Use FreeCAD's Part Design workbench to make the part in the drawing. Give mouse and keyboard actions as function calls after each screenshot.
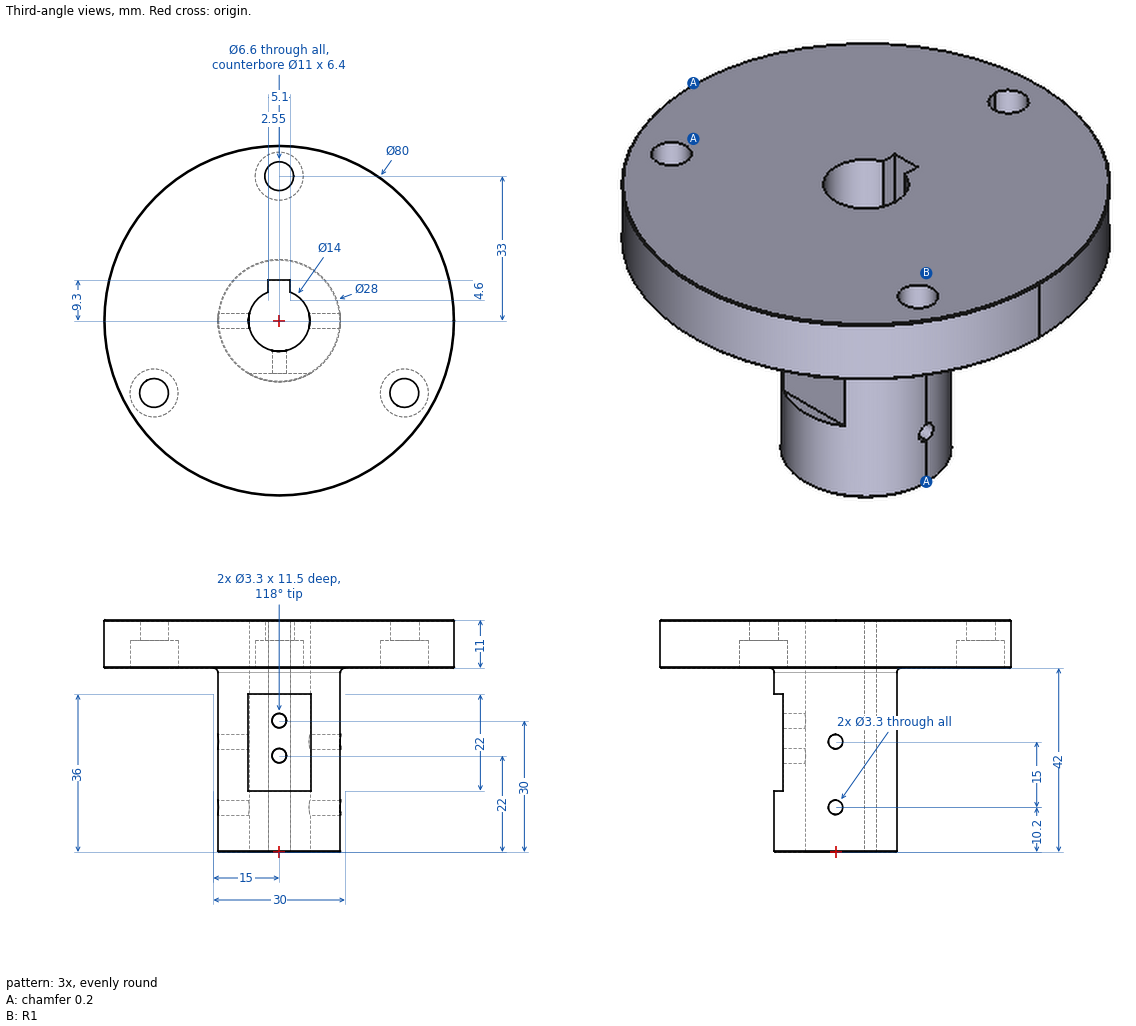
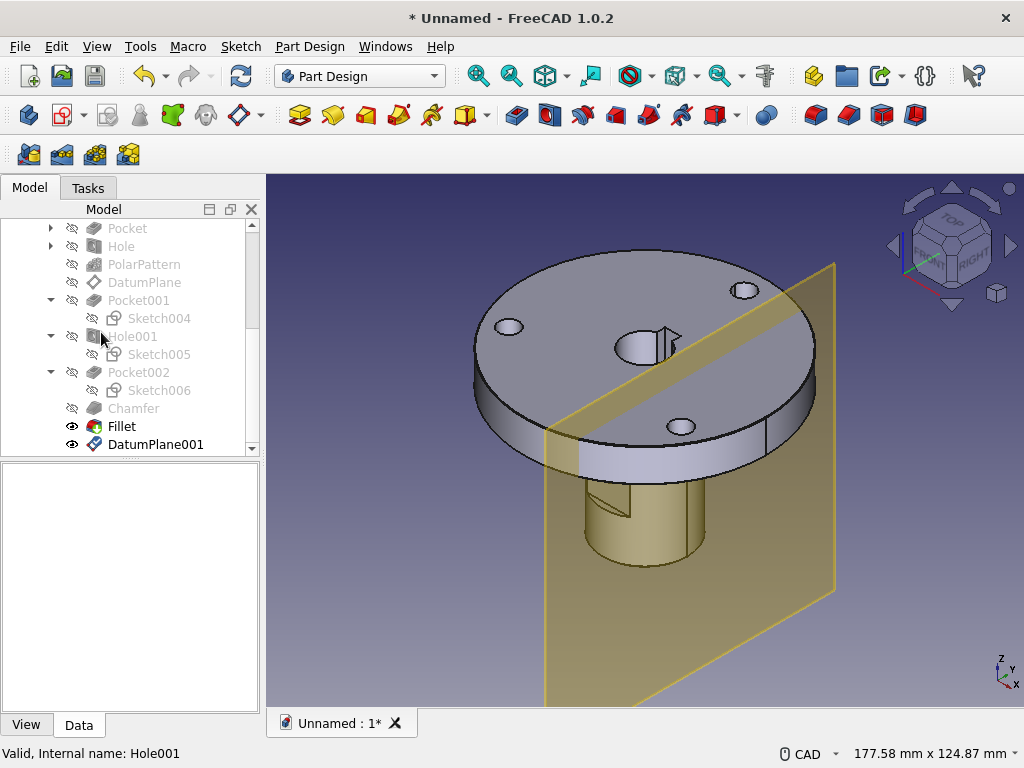
click(117, 444)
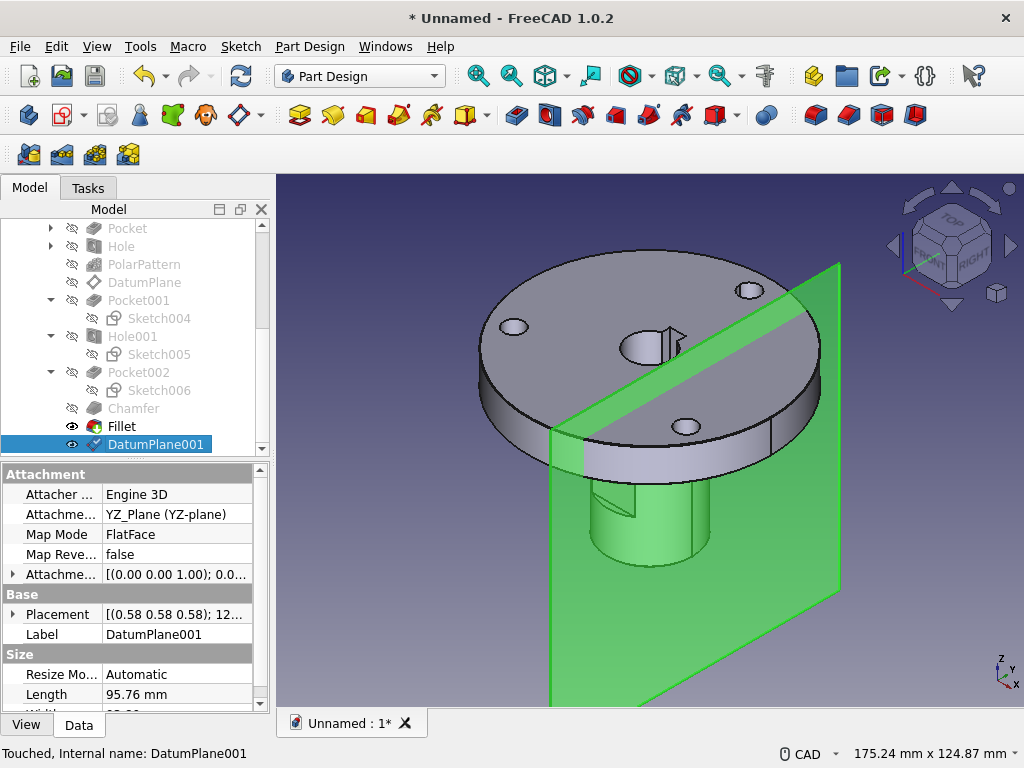
click(62, 116)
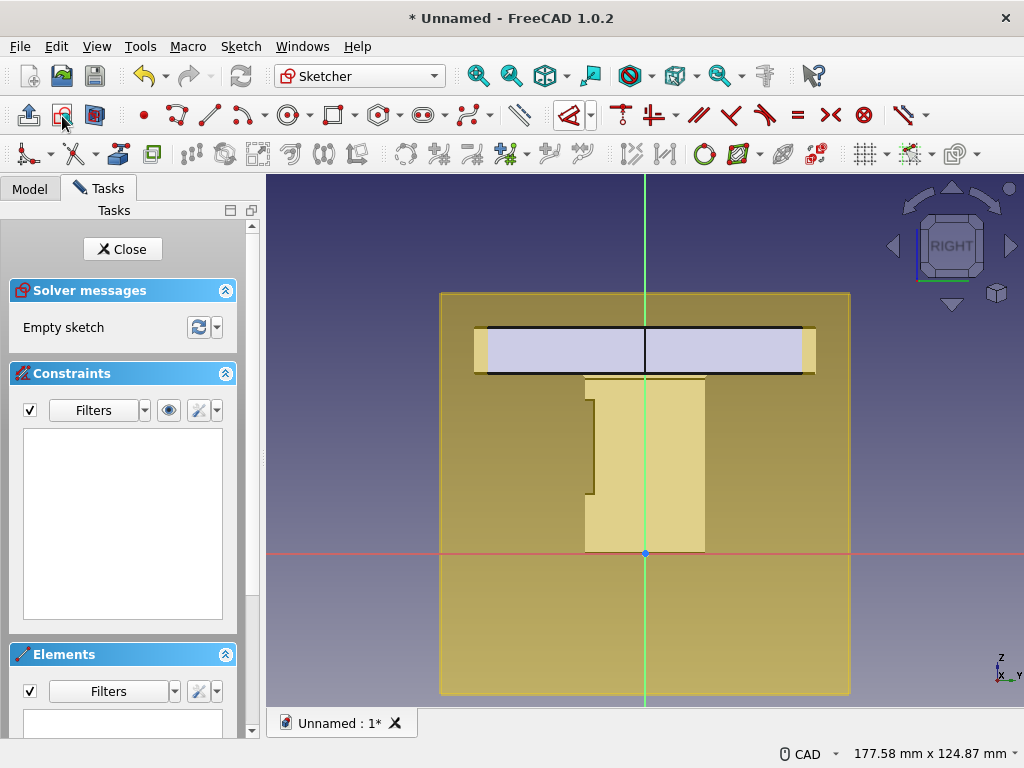
key(q)
key(s)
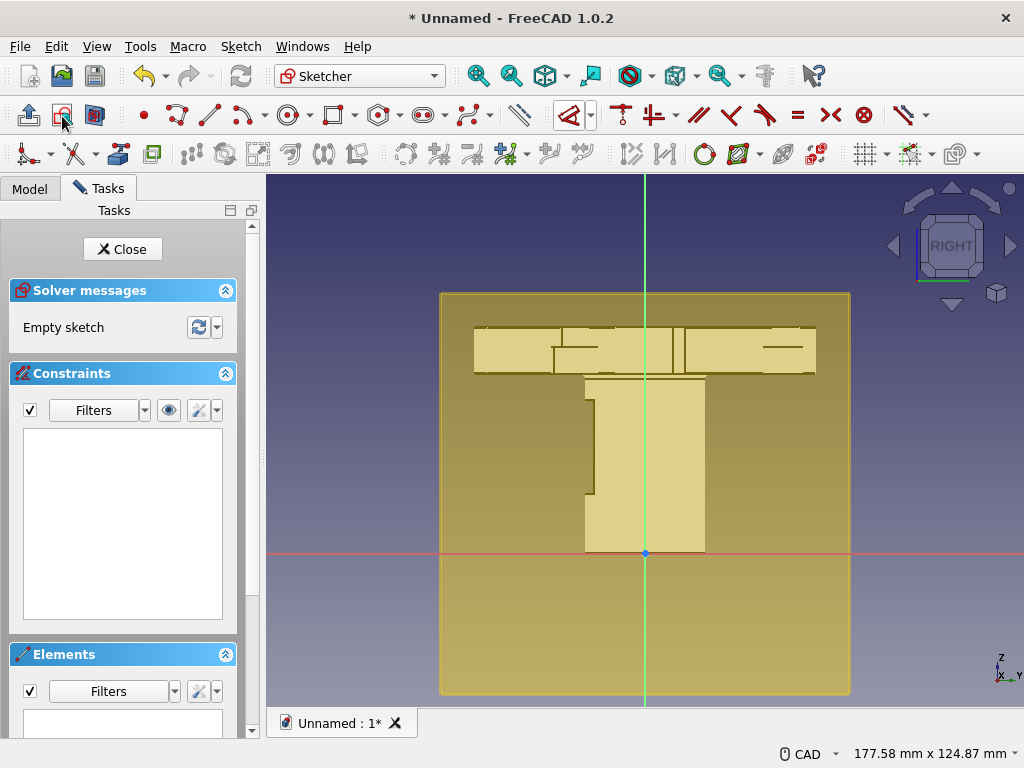
scroll(685, 529, up, 5)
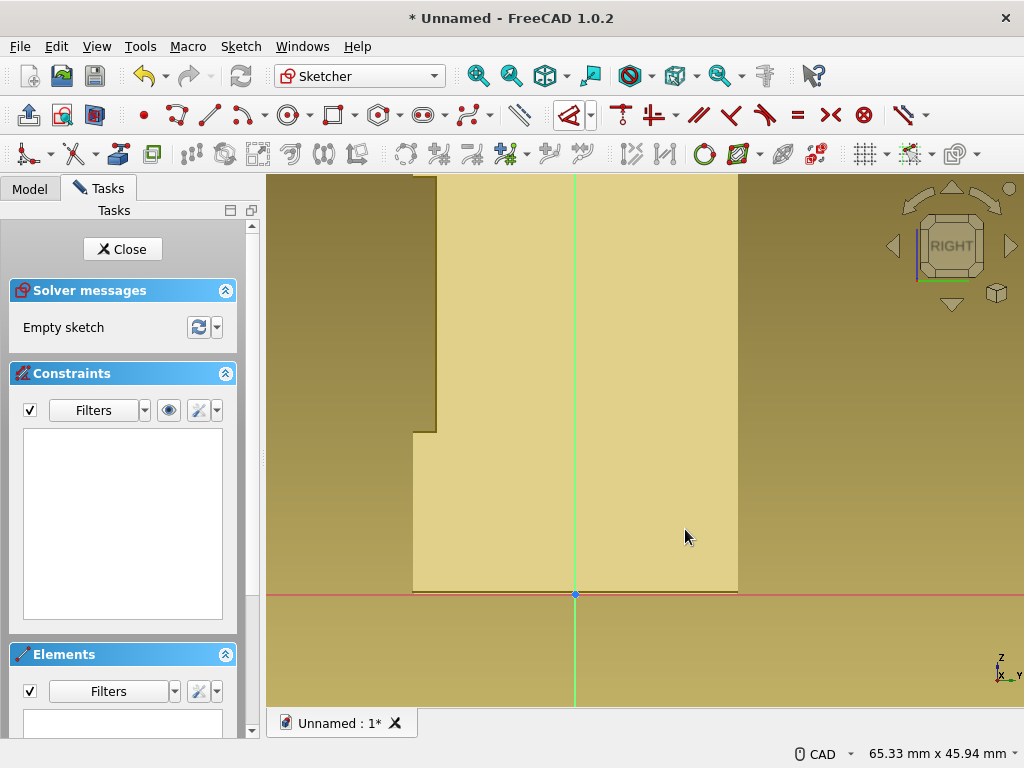
click(288, 116)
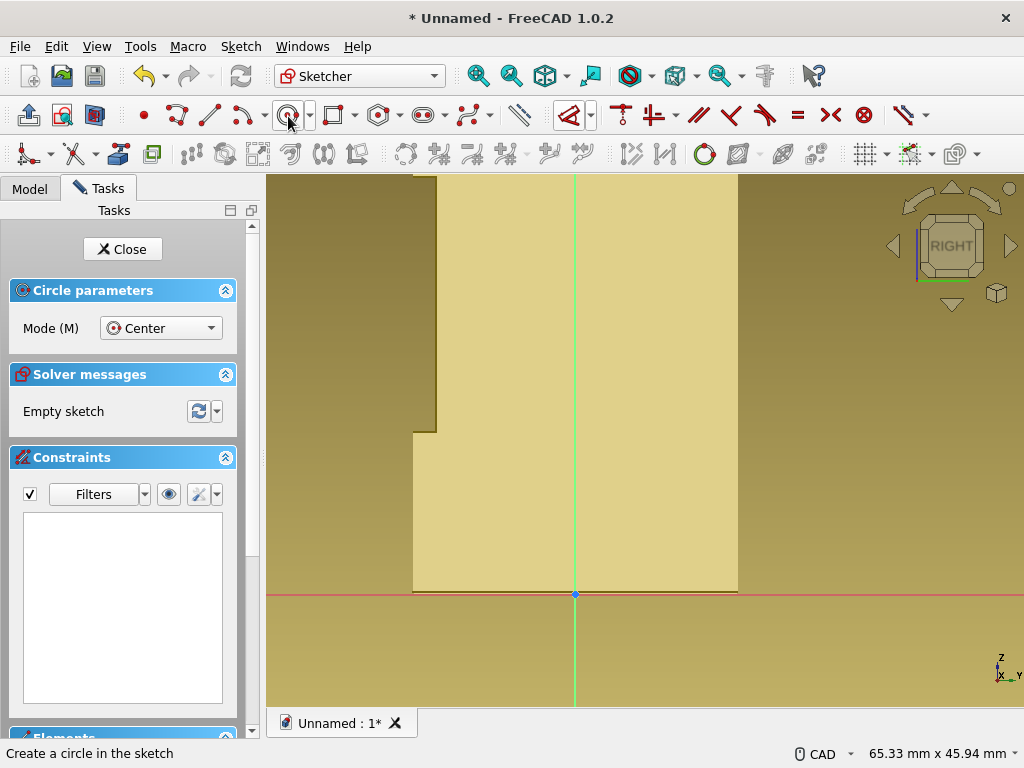
click(575, 476)
move(593, 470)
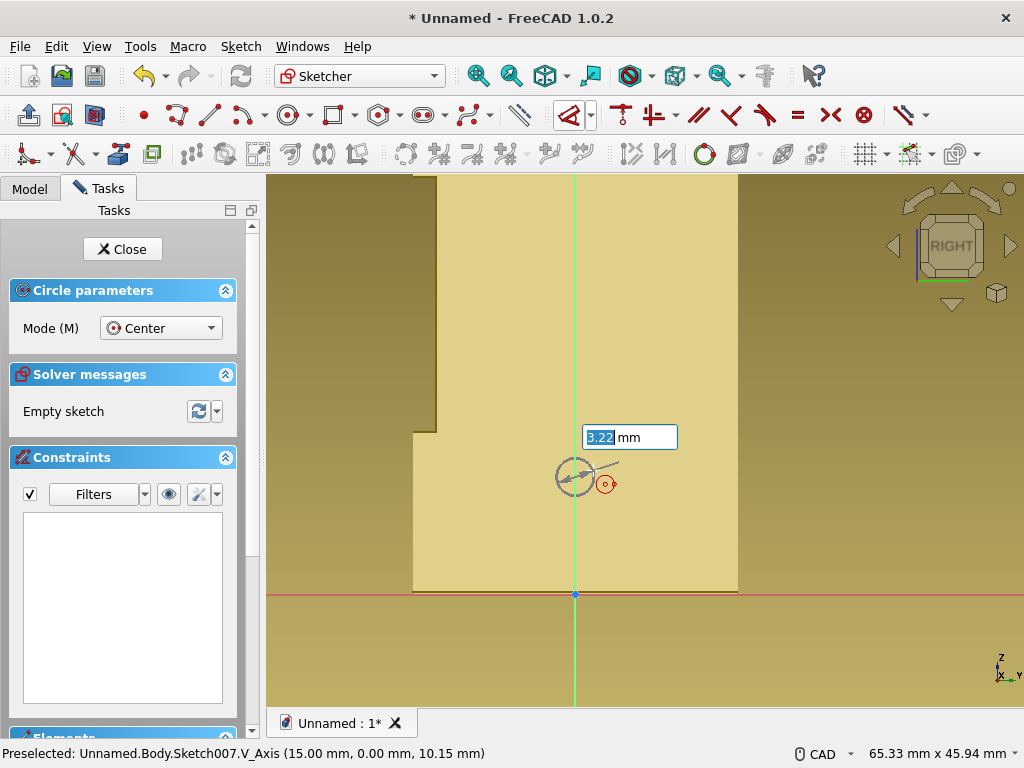
text(3.3)
key(Return)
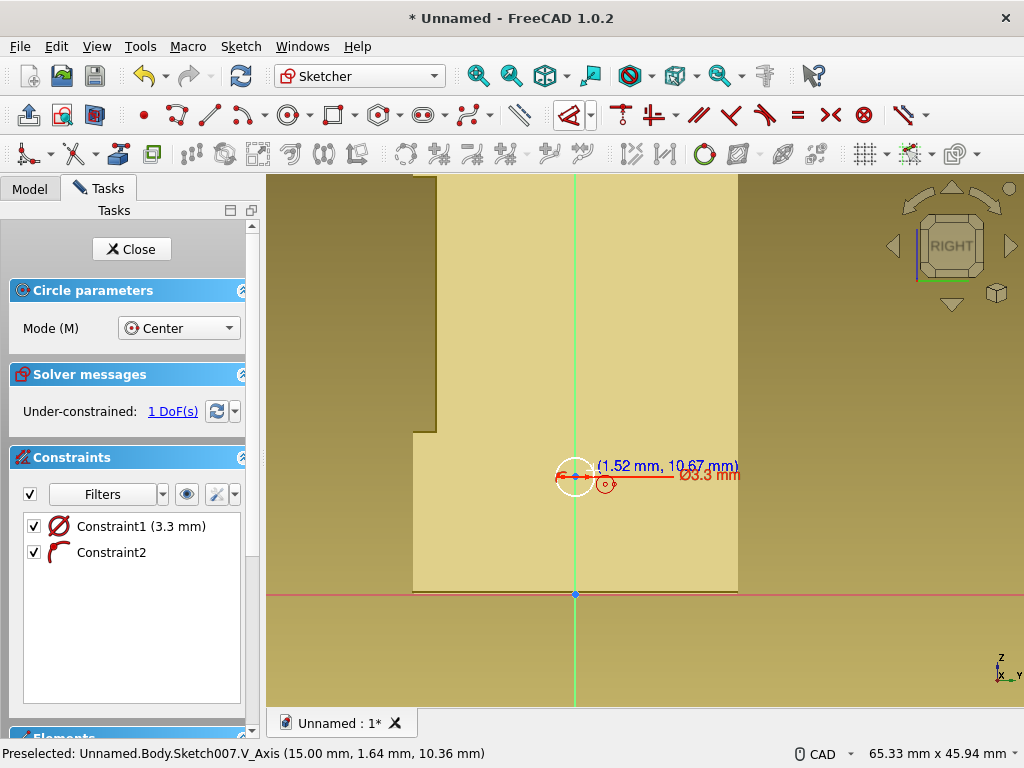
click(575, 302)
move(593, 296)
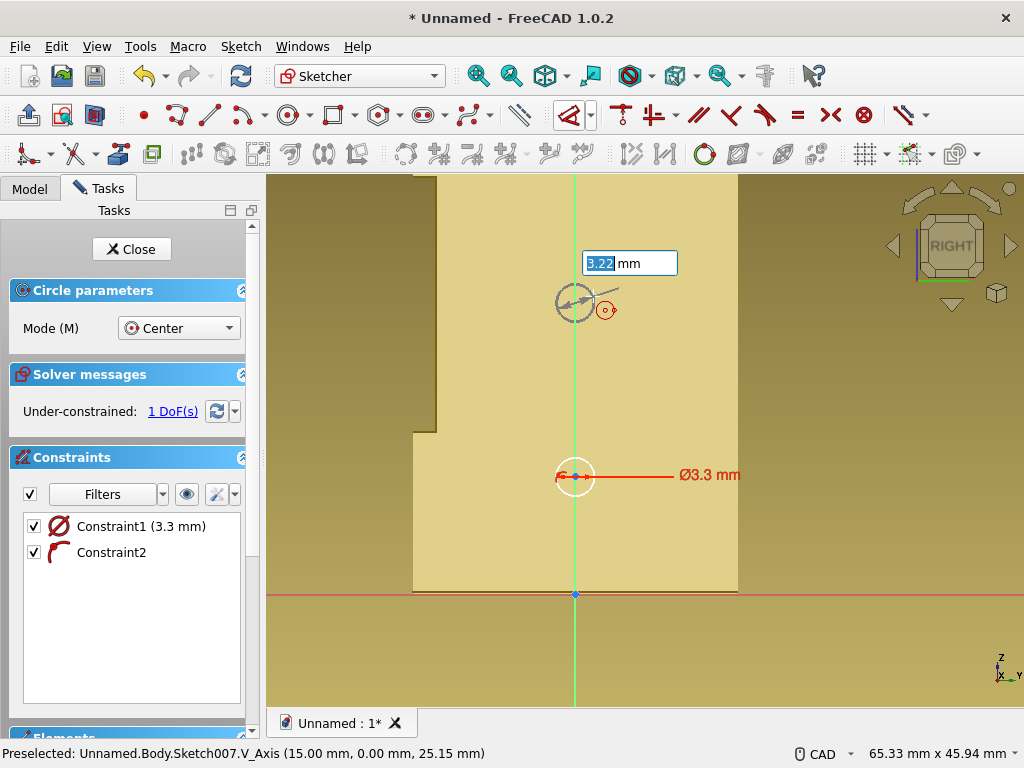
text(3.3)
key(Return)
key(Escape)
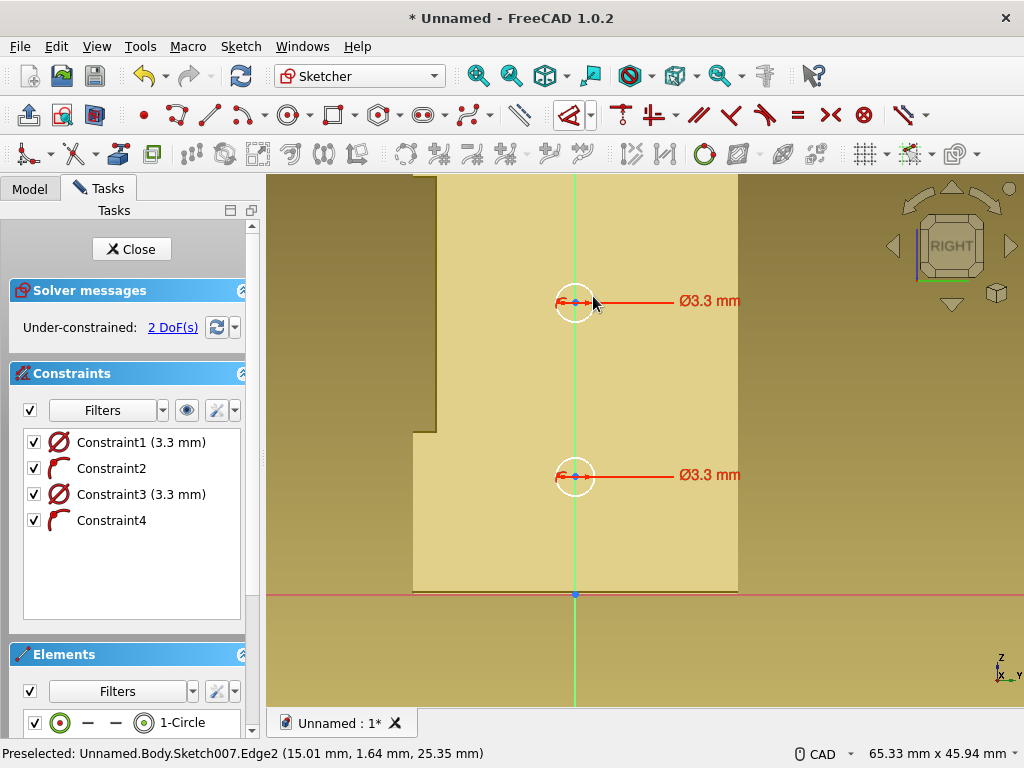
click(575, 477)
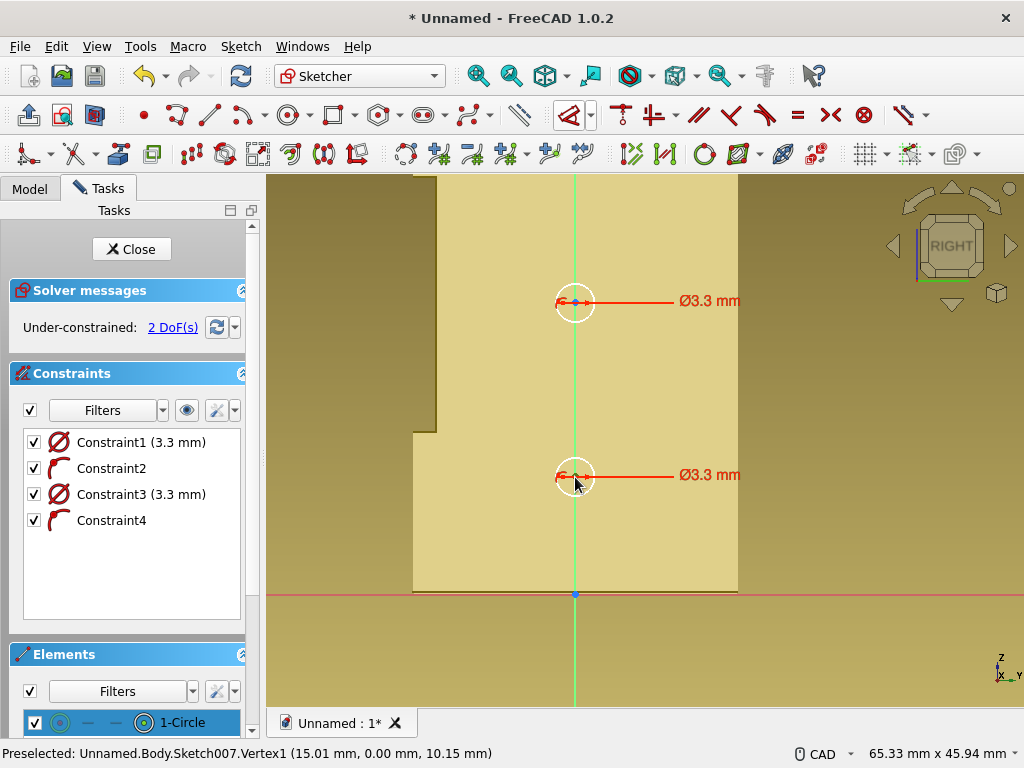
click(575, 303)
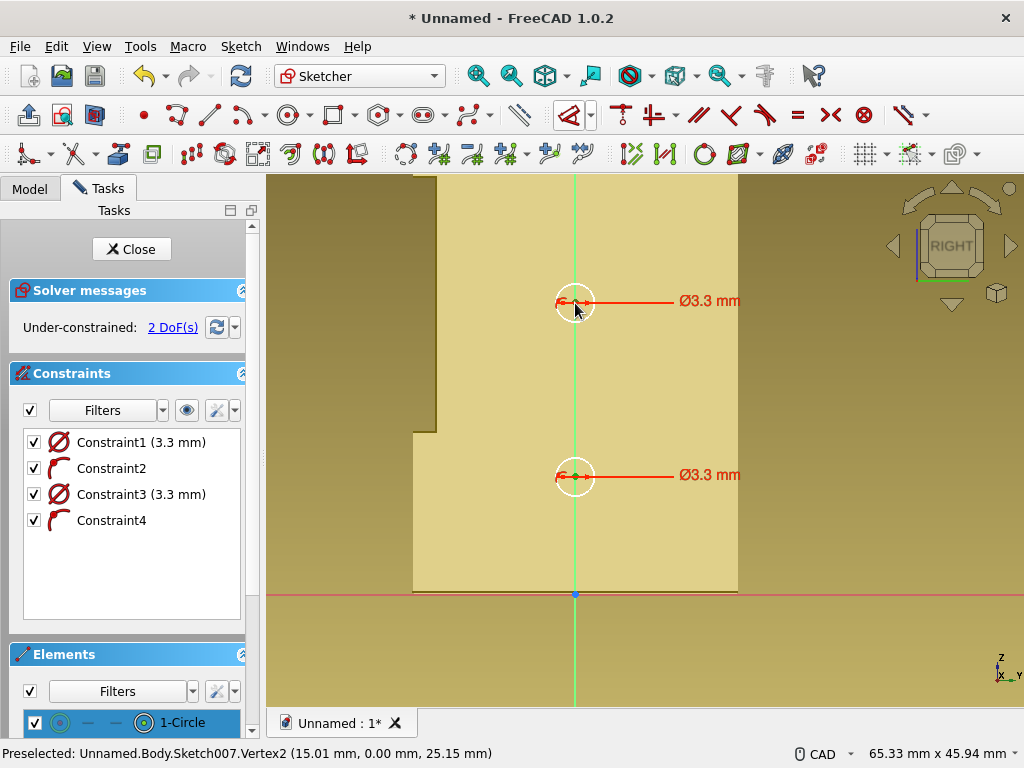
key(i)